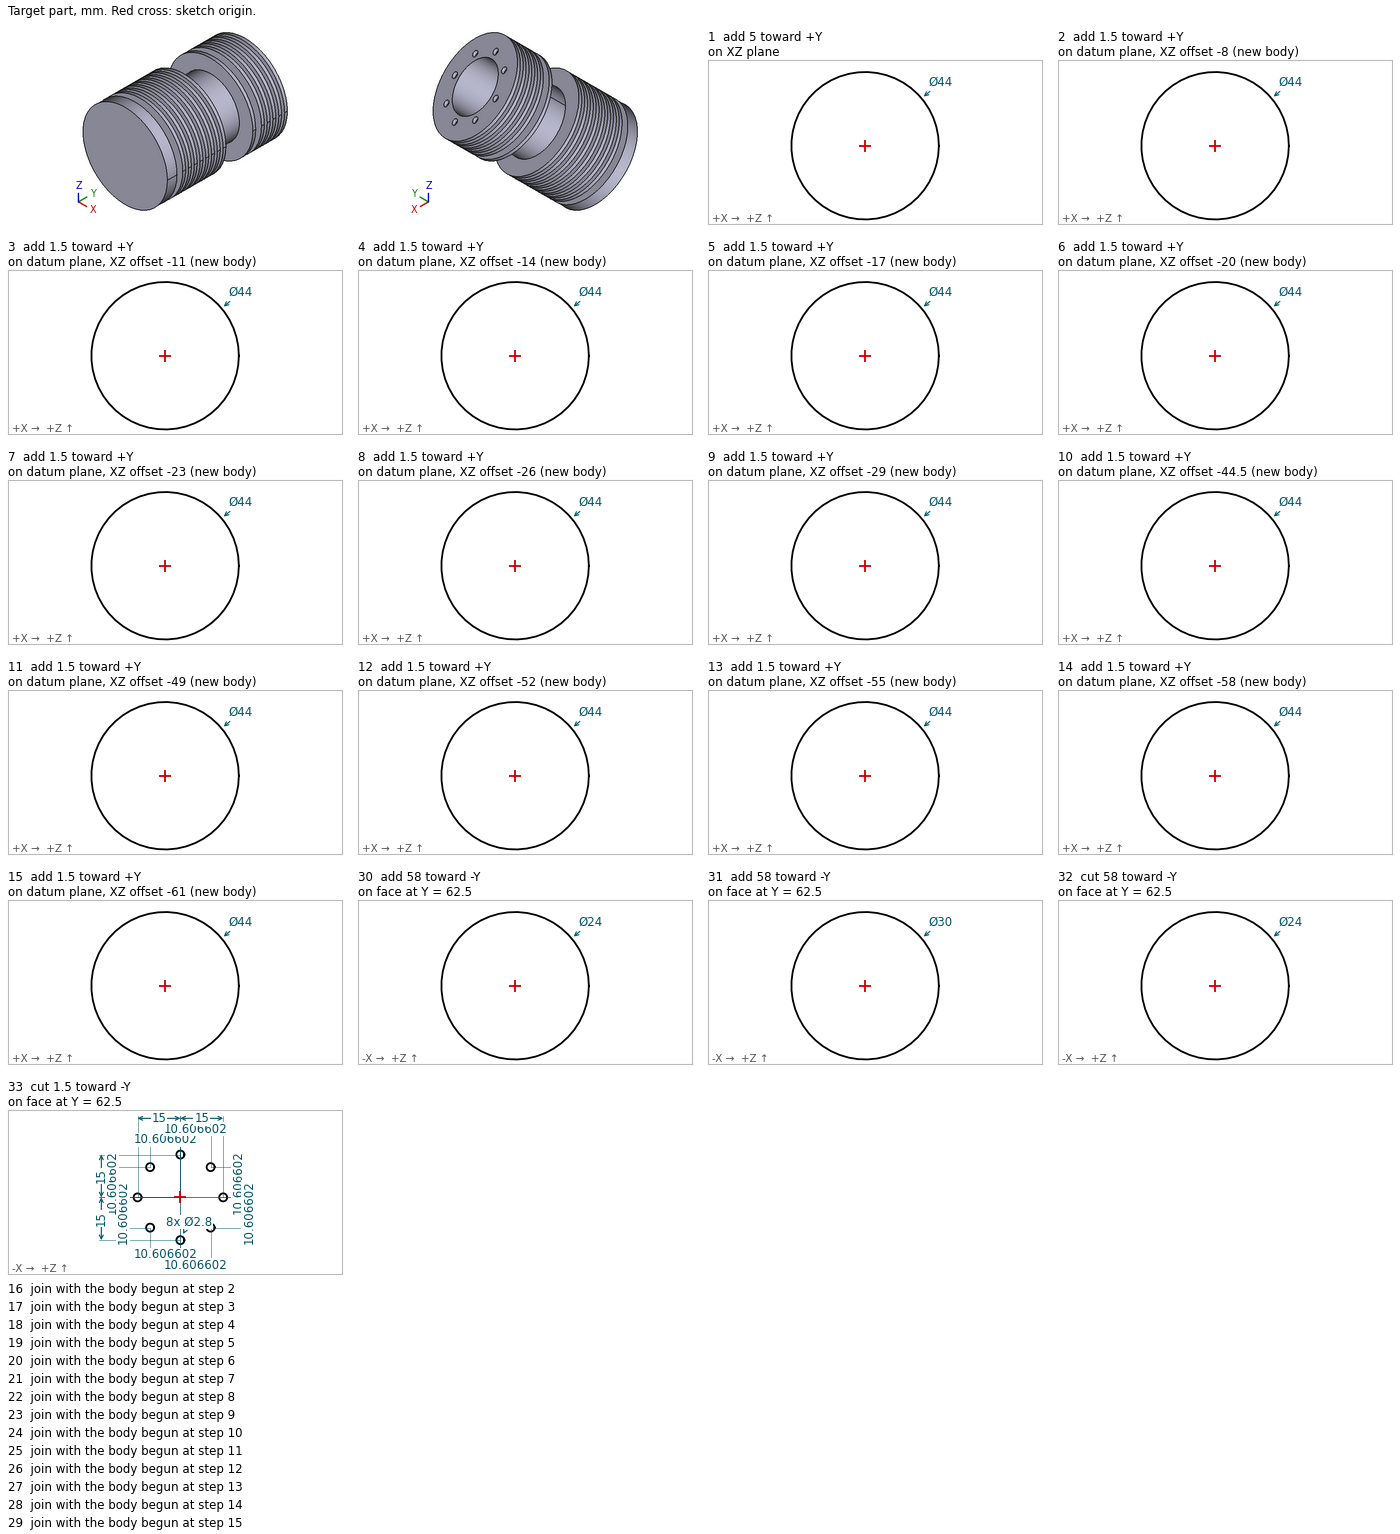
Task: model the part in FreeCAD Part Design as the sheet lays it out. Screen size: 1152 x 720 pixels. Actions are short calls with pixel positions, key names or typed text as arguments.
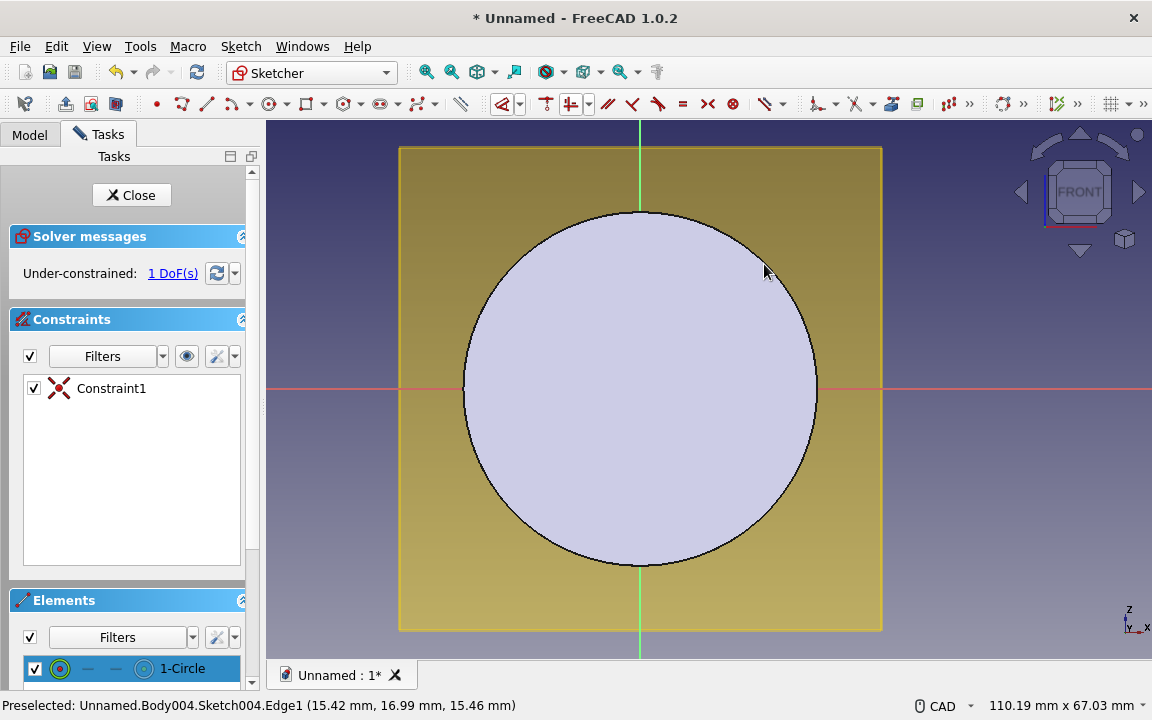
key(k)
key(o)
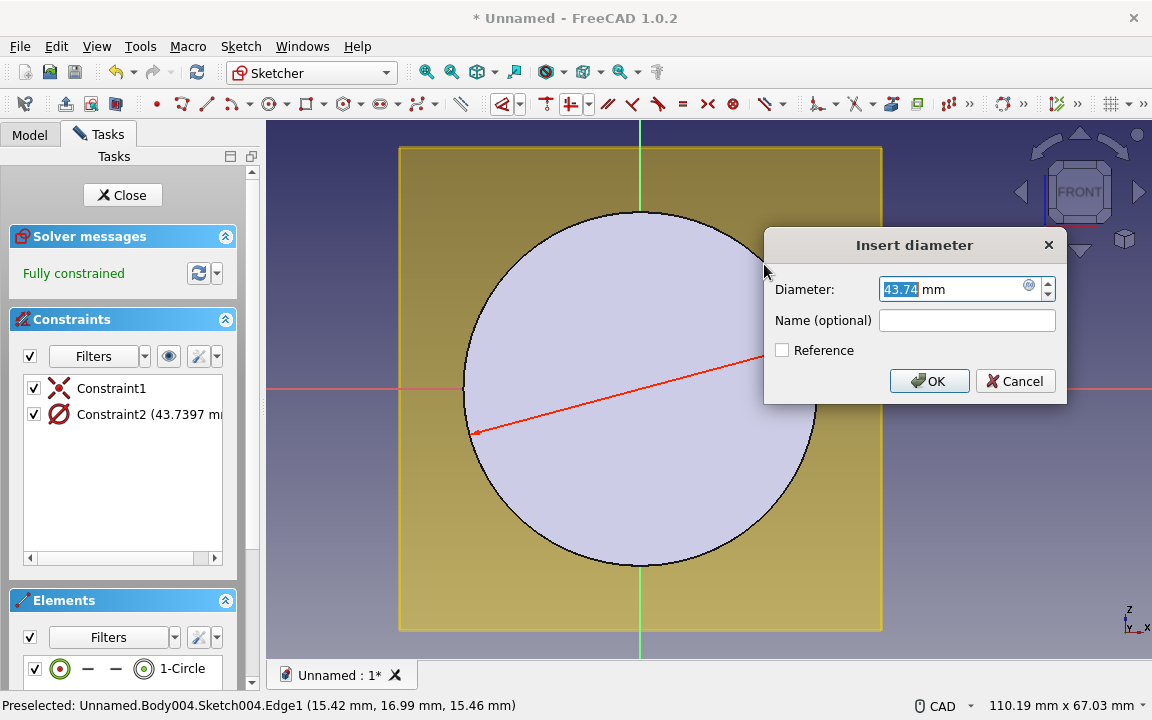
text(44)
key(Return)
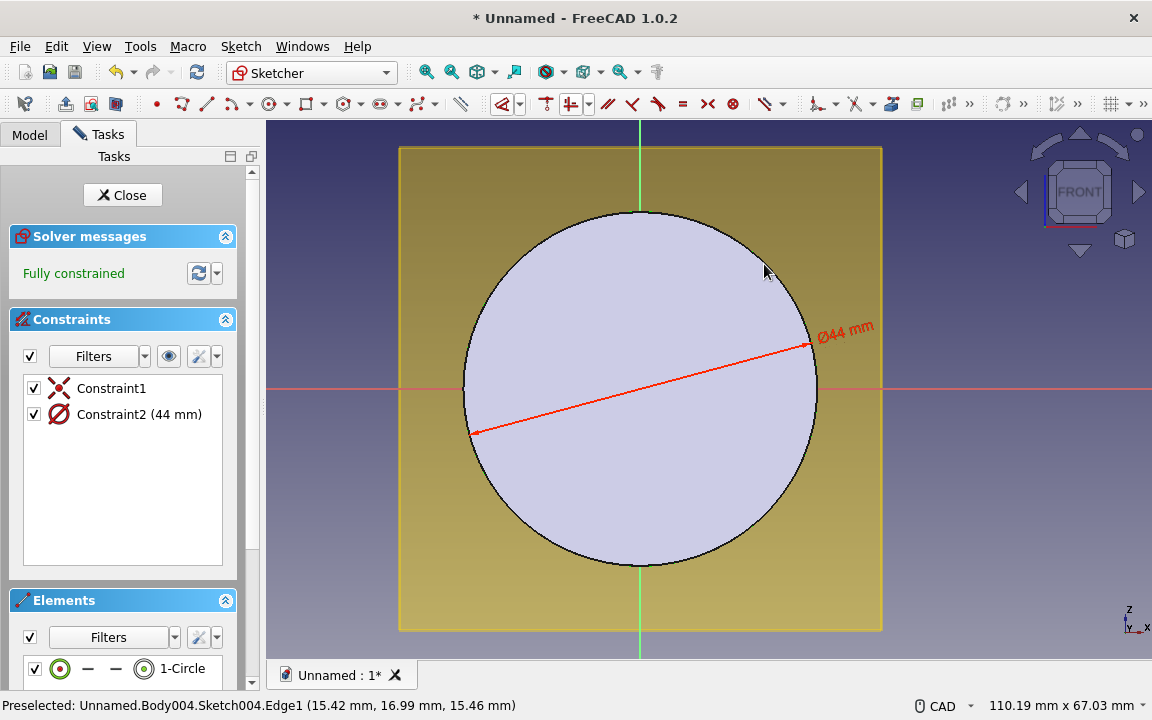
click(123, 195)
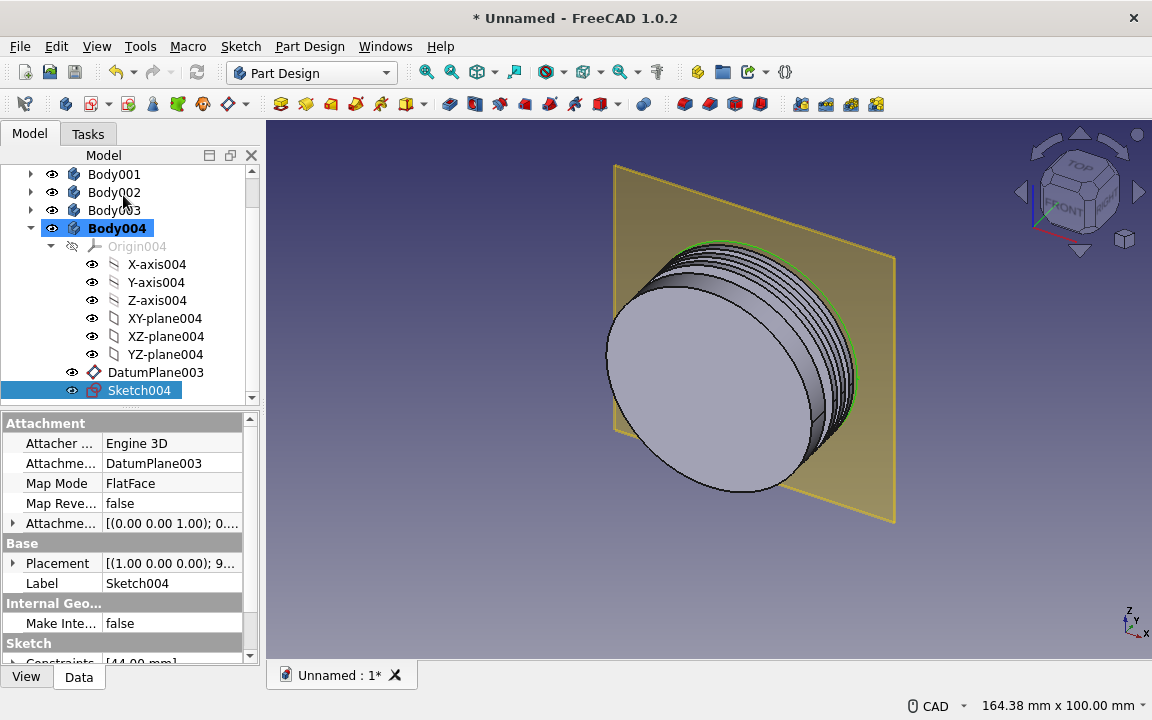
click(281, 104)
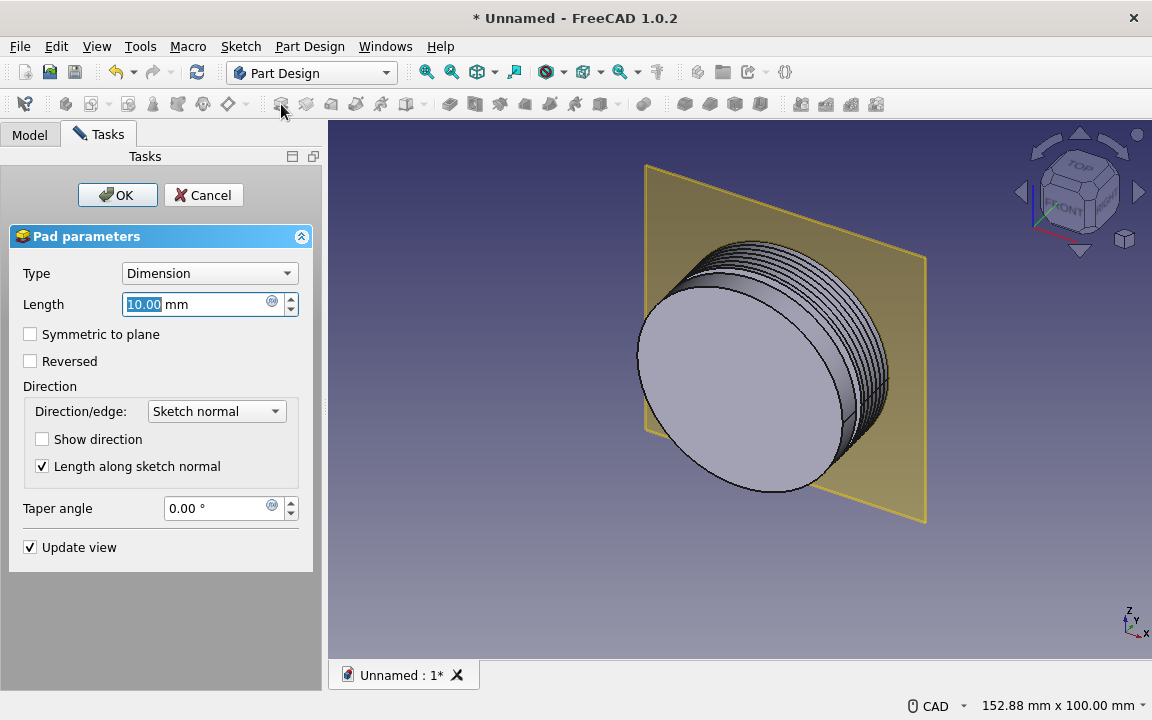
text(1.5)
key(Tab)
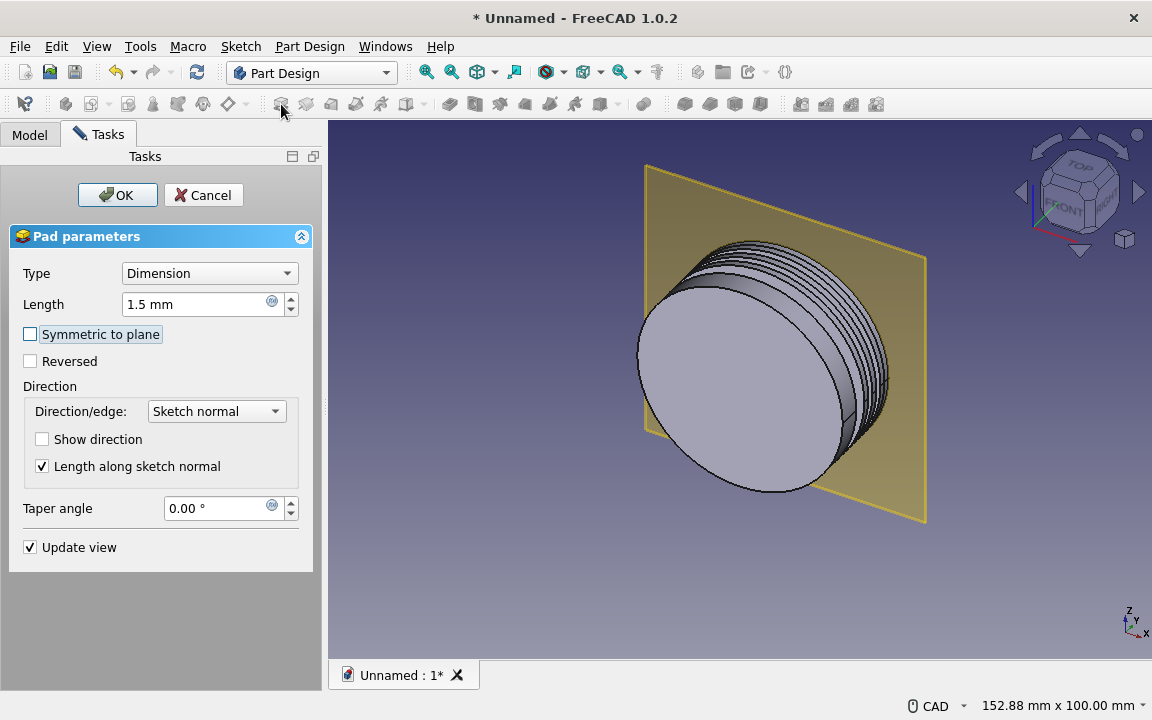
click(31, 361)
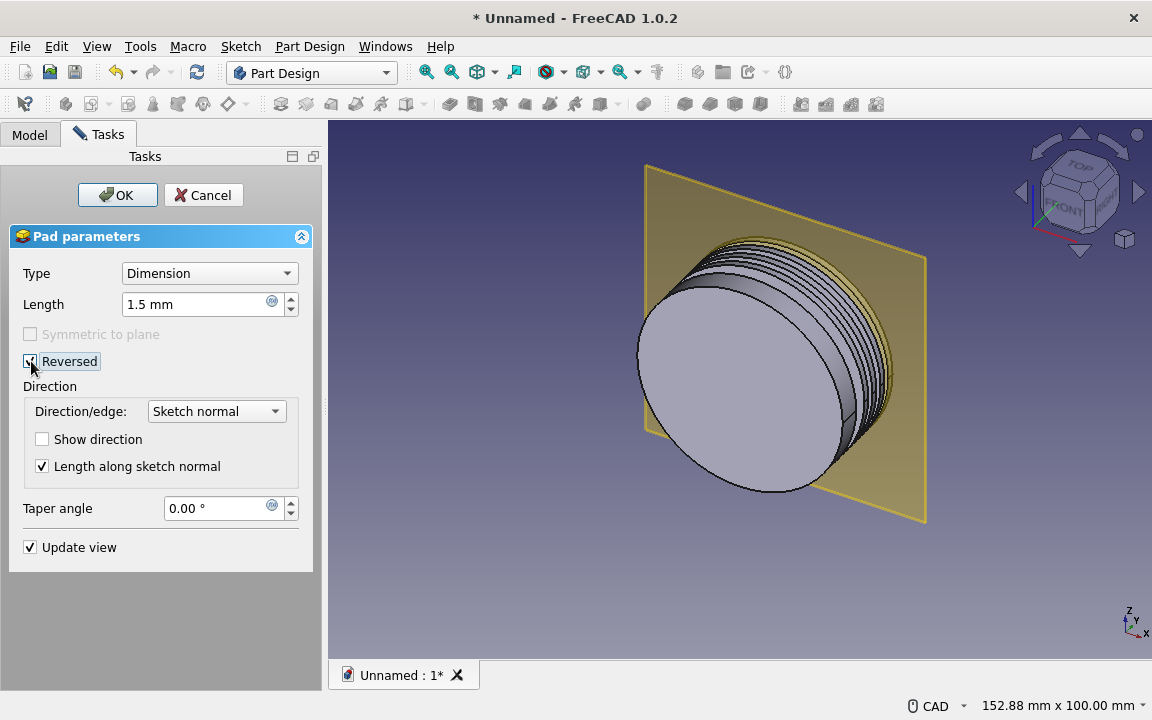
click(118, 195)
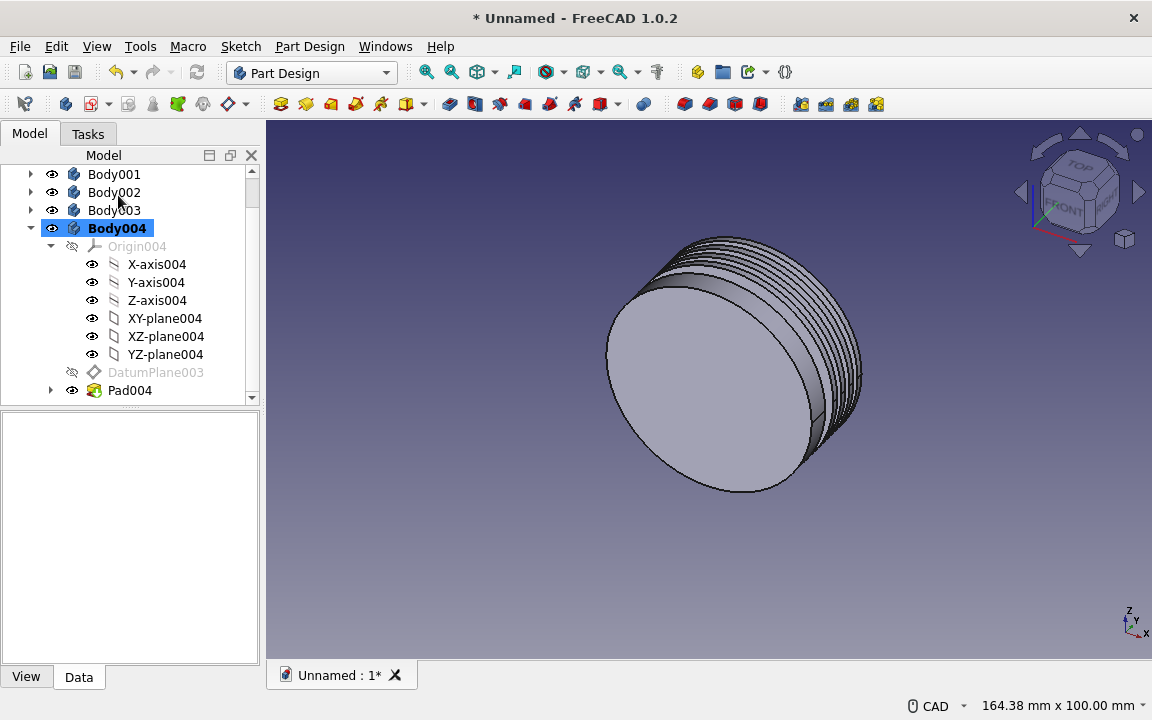
click(66, 104)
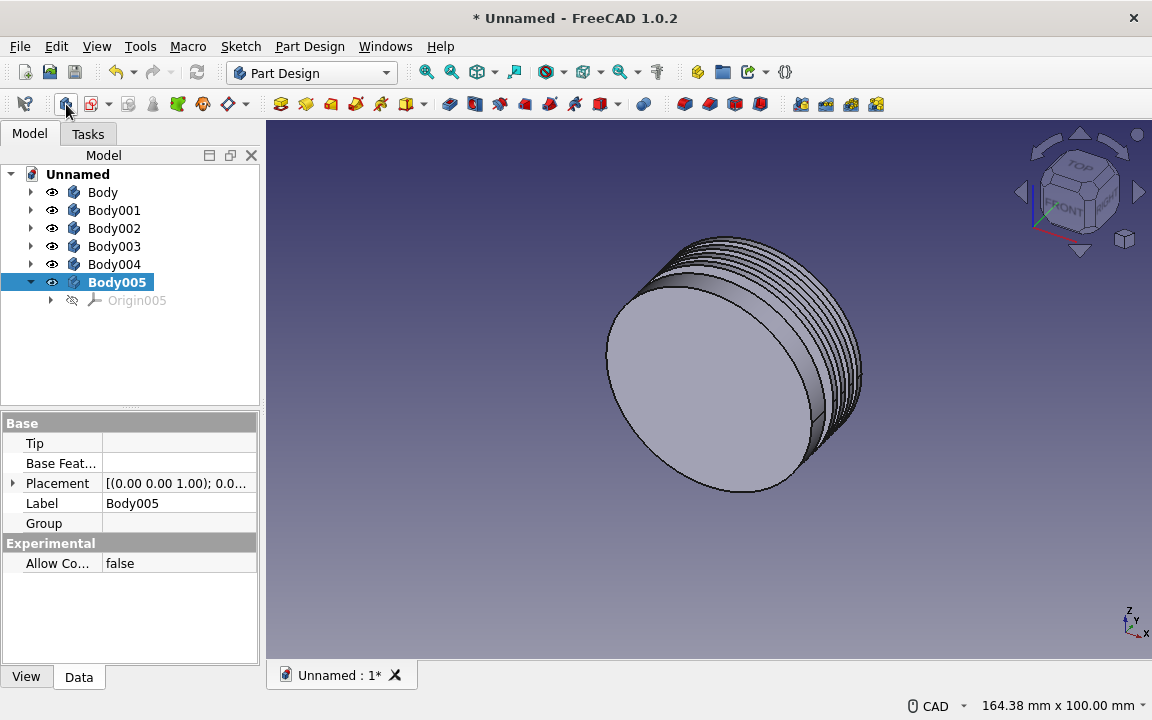
click(51, 300)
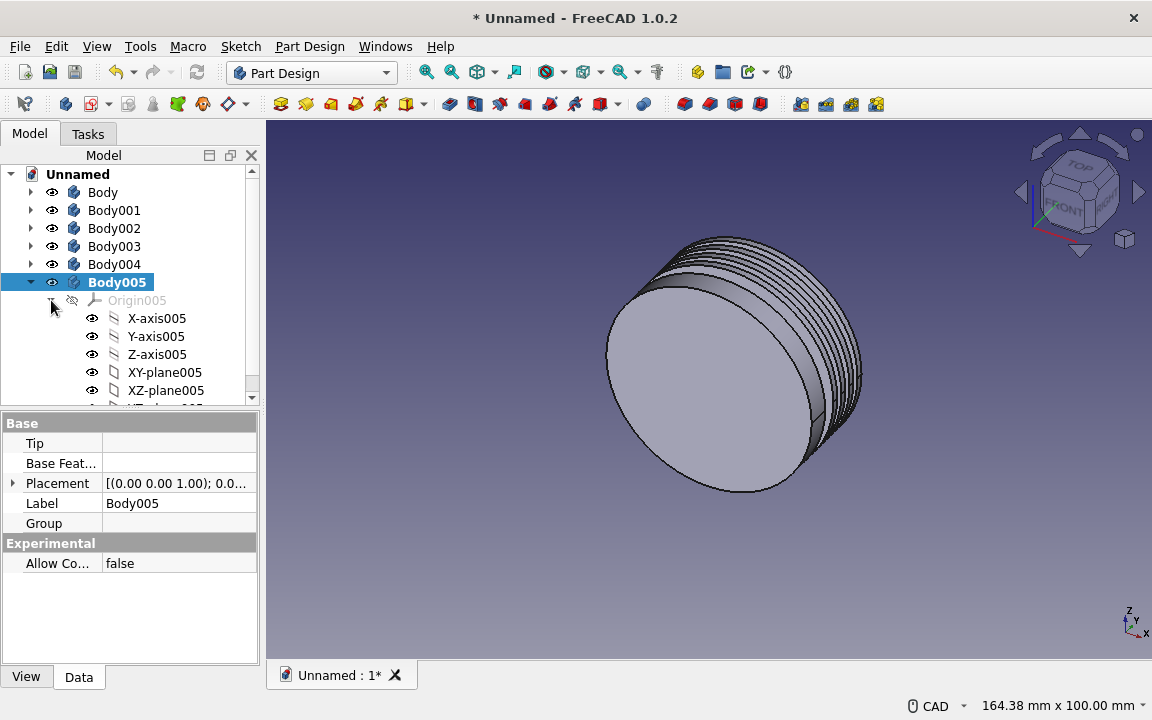
click(137, 390)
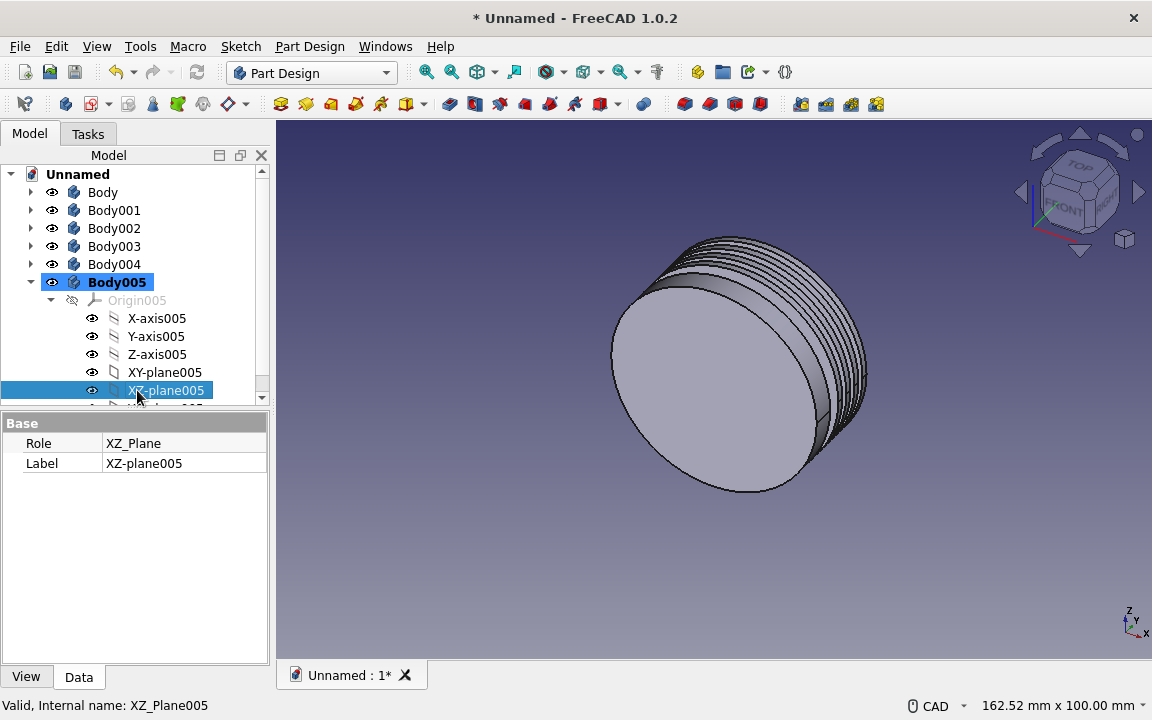
click(228, 104)